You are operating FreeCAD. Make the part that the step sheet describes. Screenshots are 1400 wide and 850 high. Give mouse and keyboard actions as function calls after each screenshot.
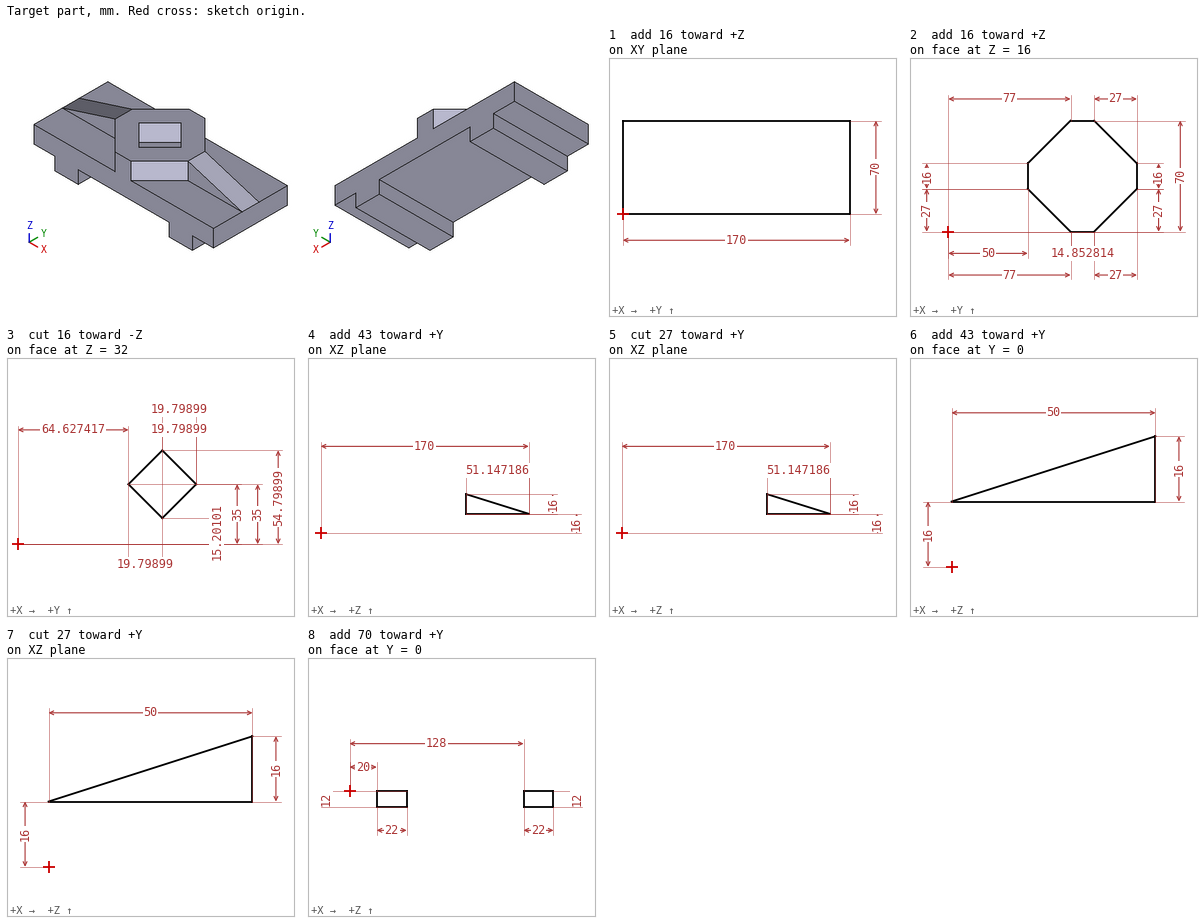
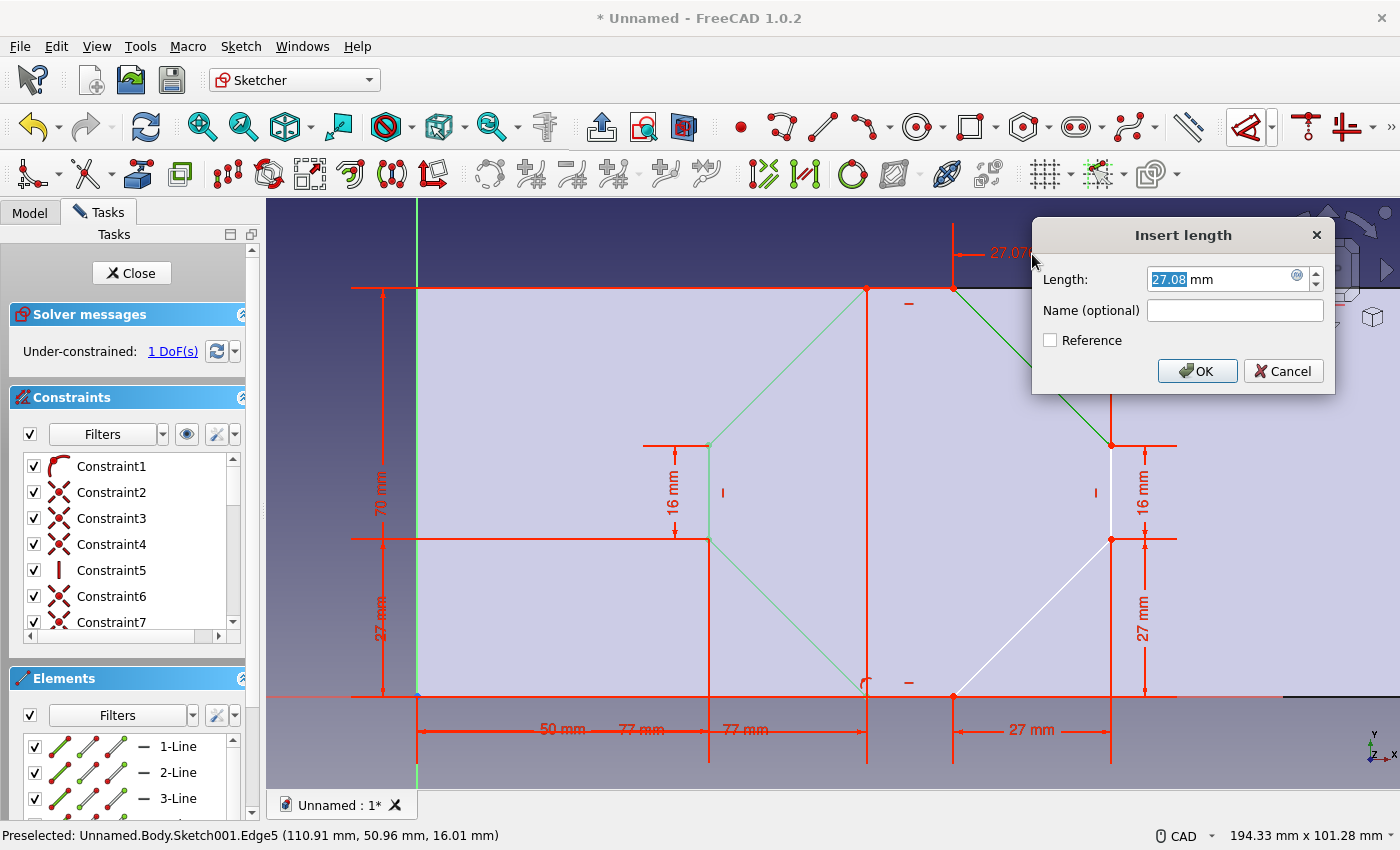
text(27)
key(Return)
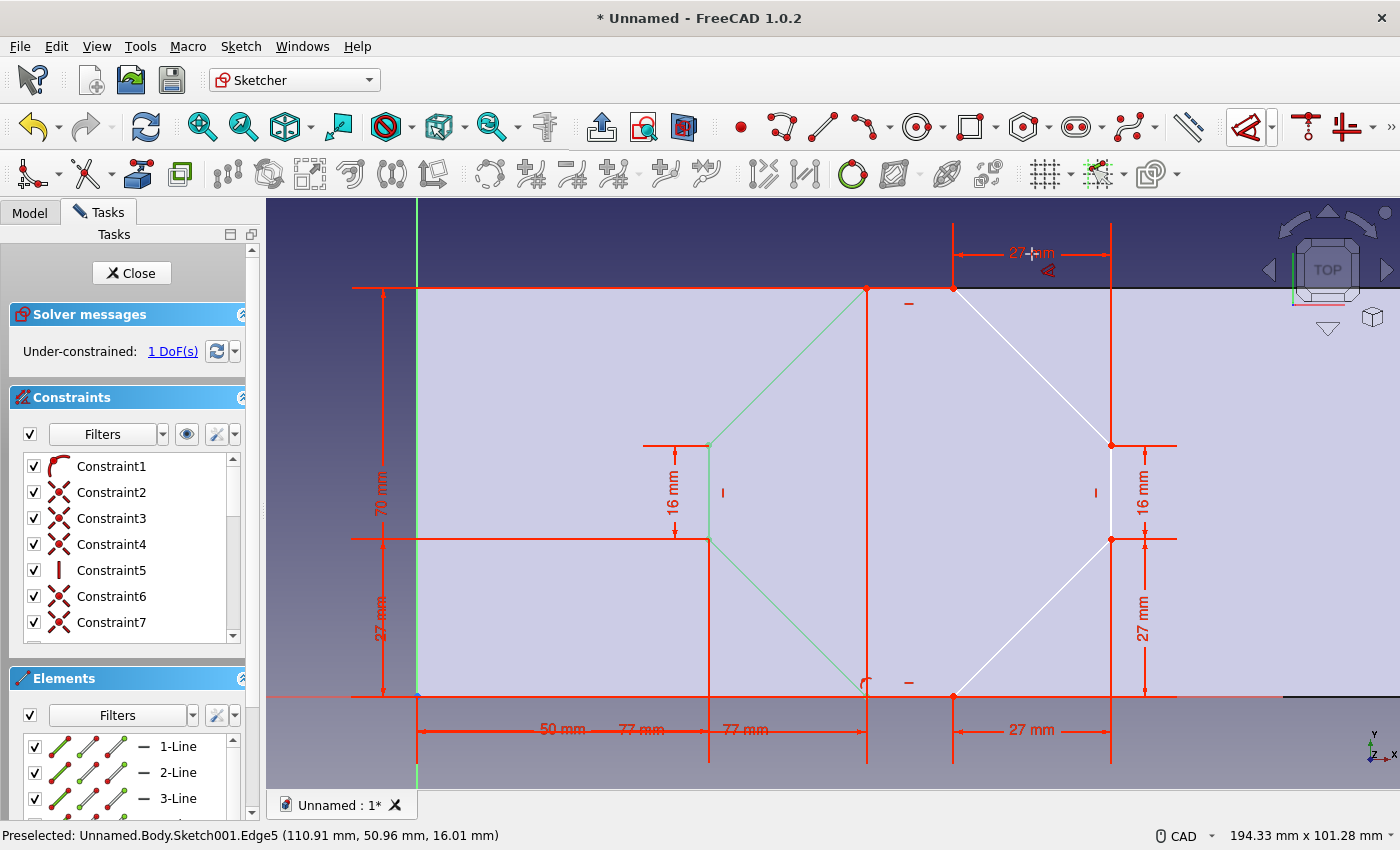
click(893, 697)
click(910, 731)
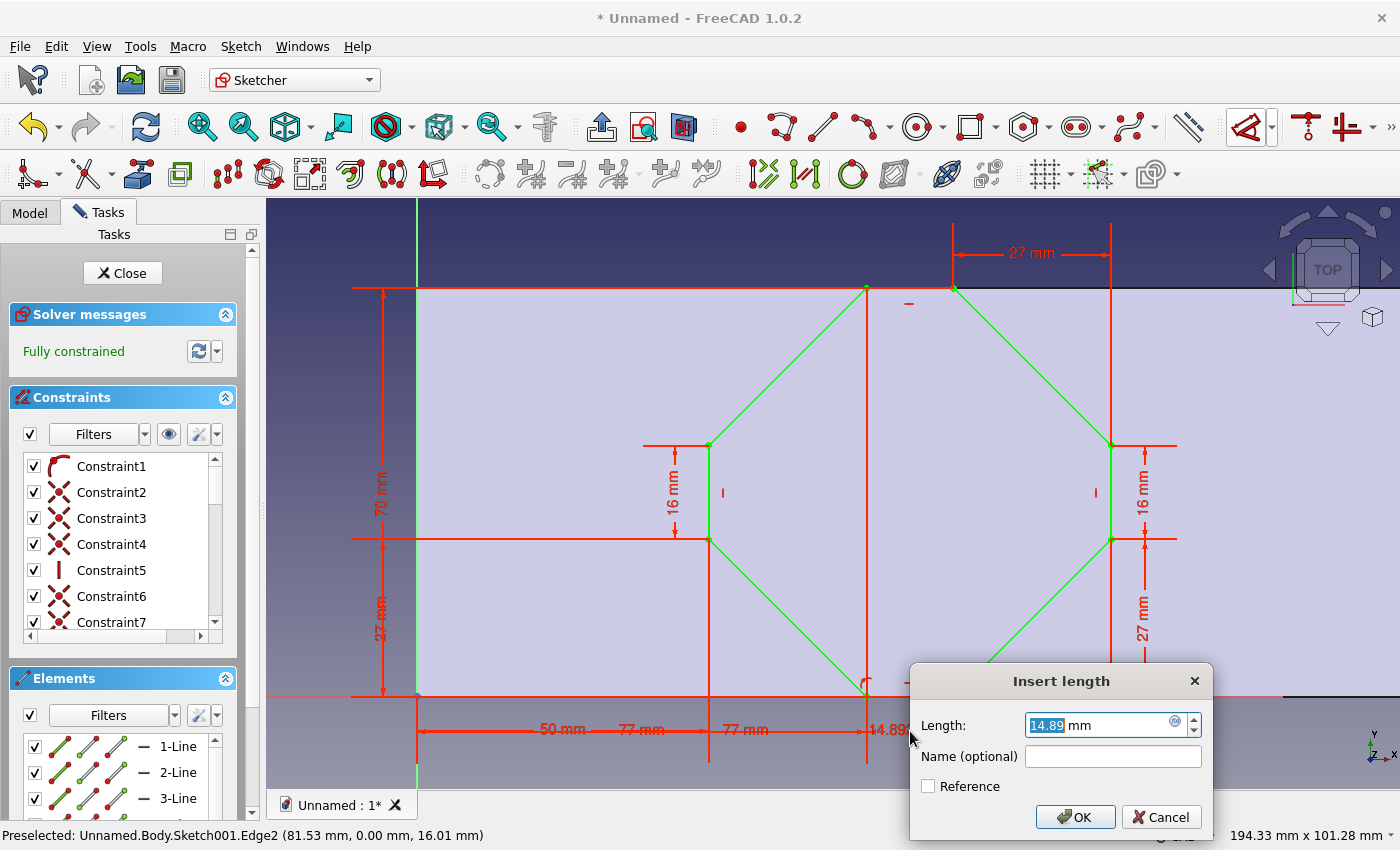
text(14.852814)
key(Return)
key(Escape)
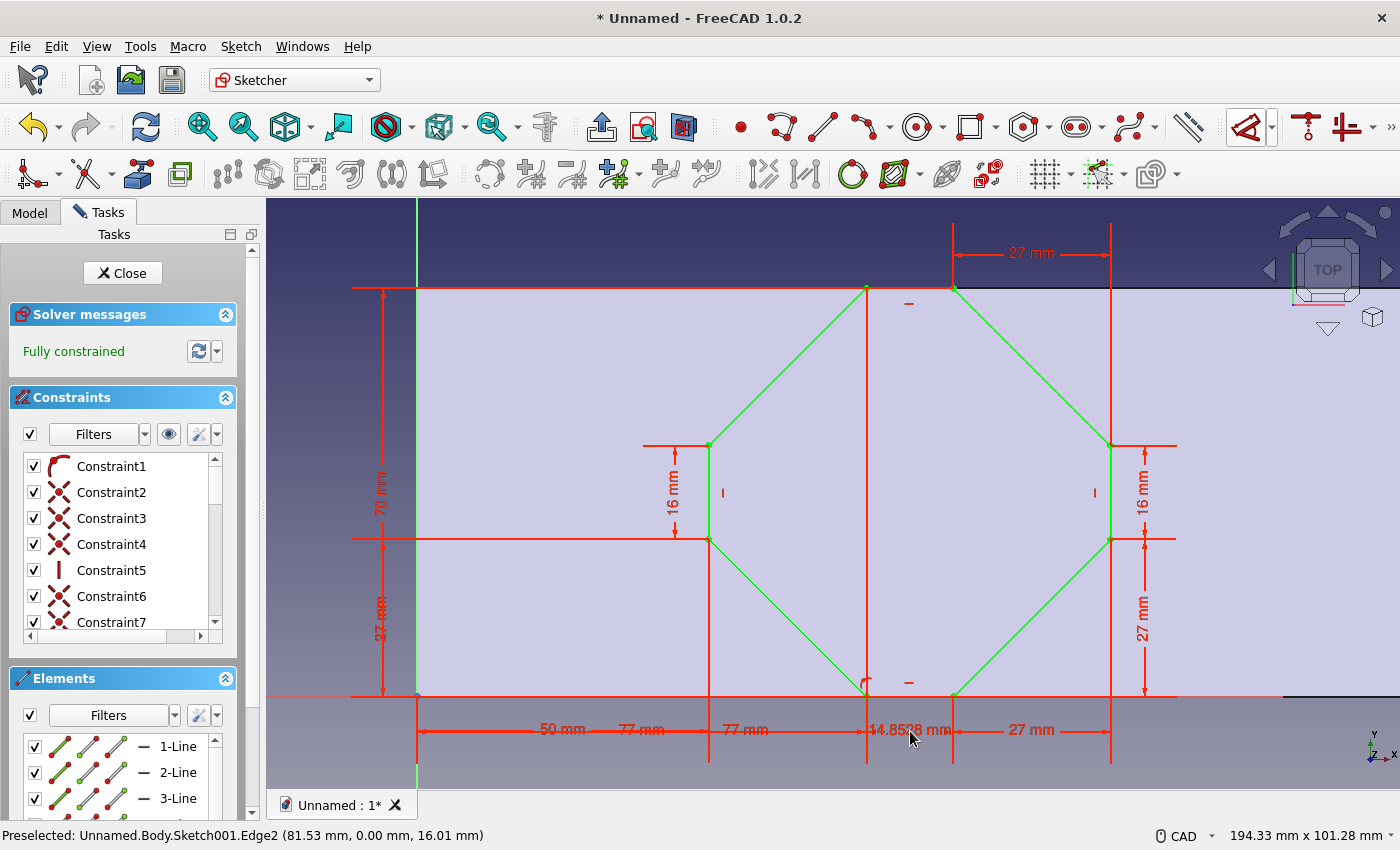
click(123, 273)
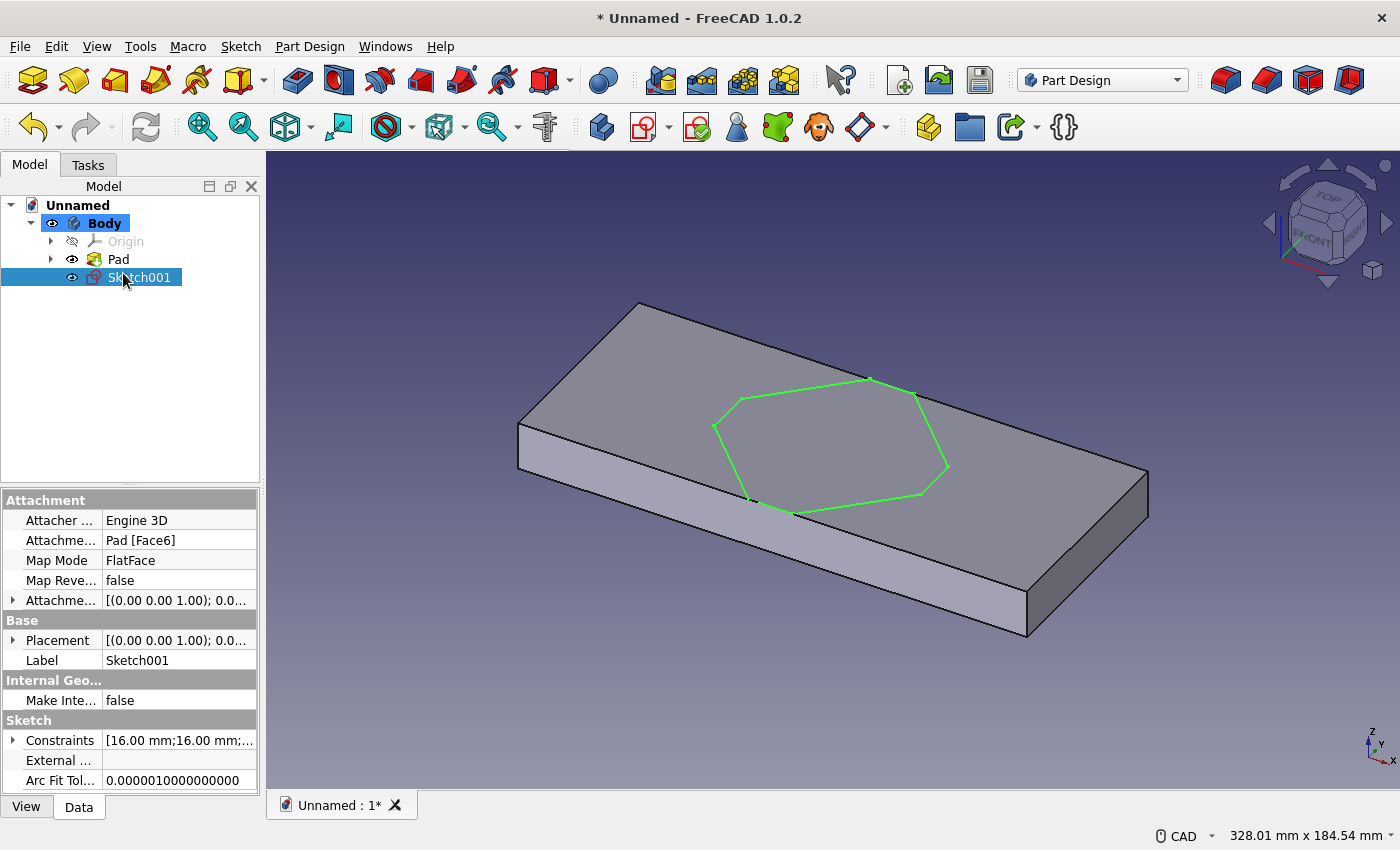
click(33, 80)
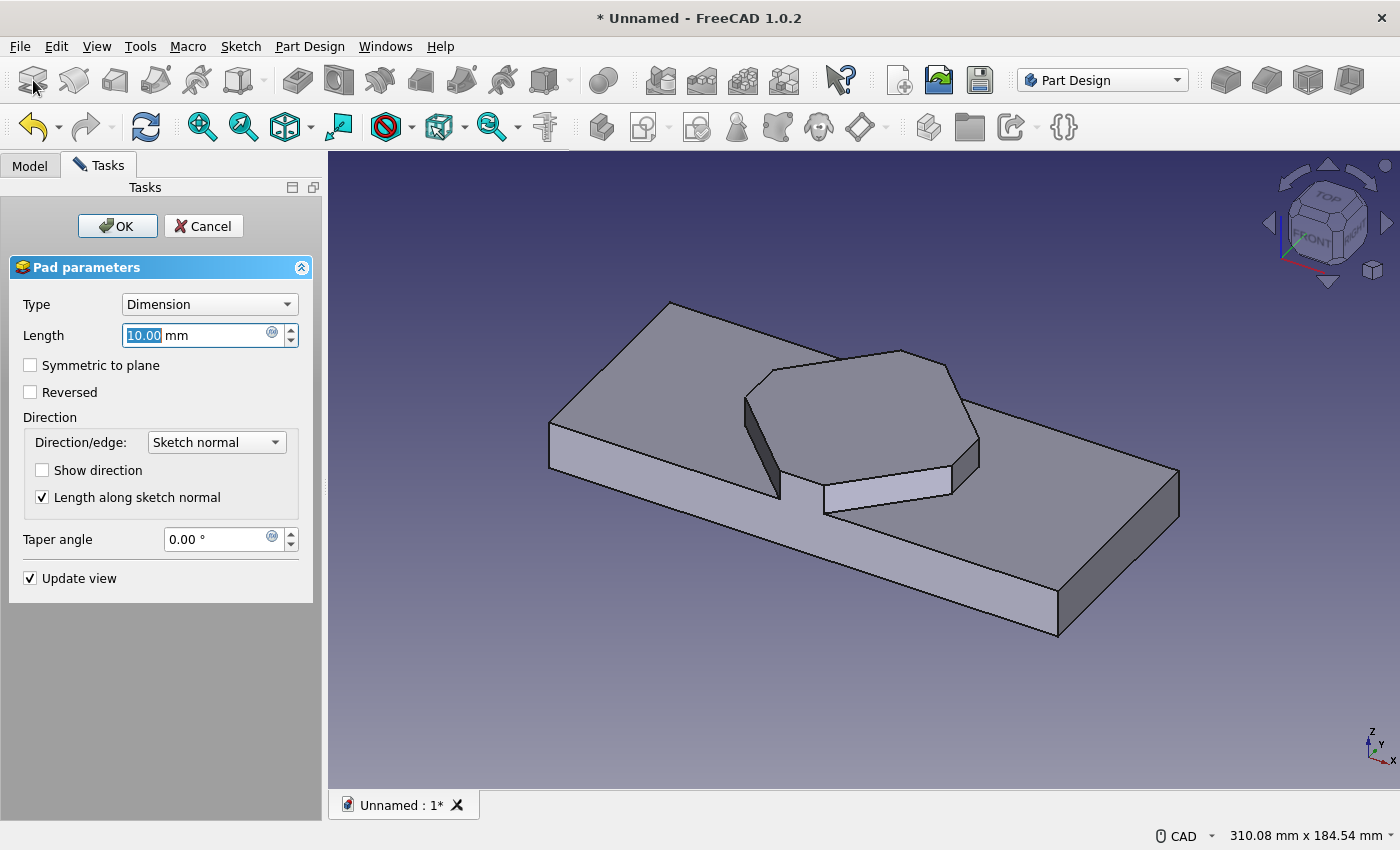
text(16)
key(Tab)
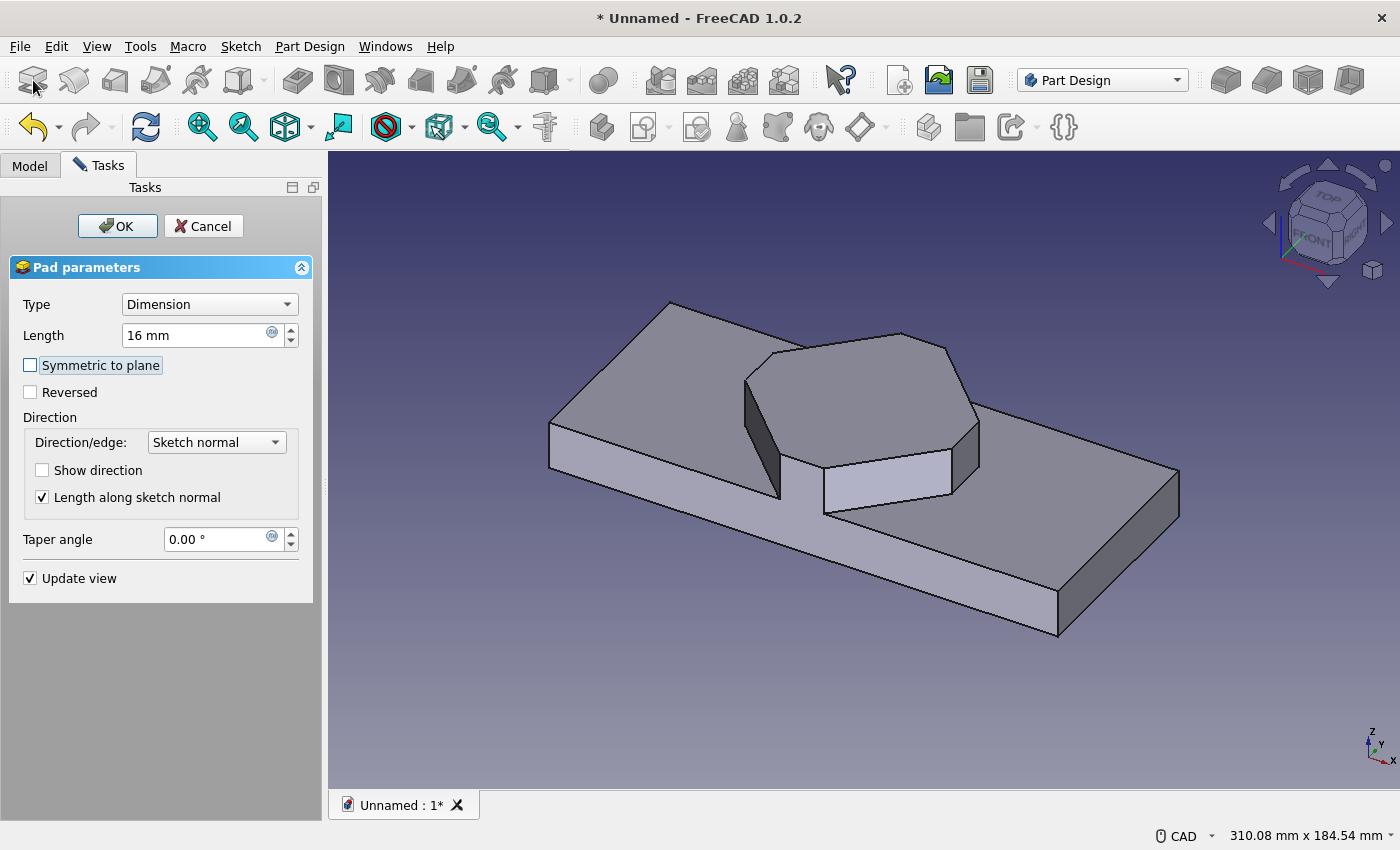
click(118, 226)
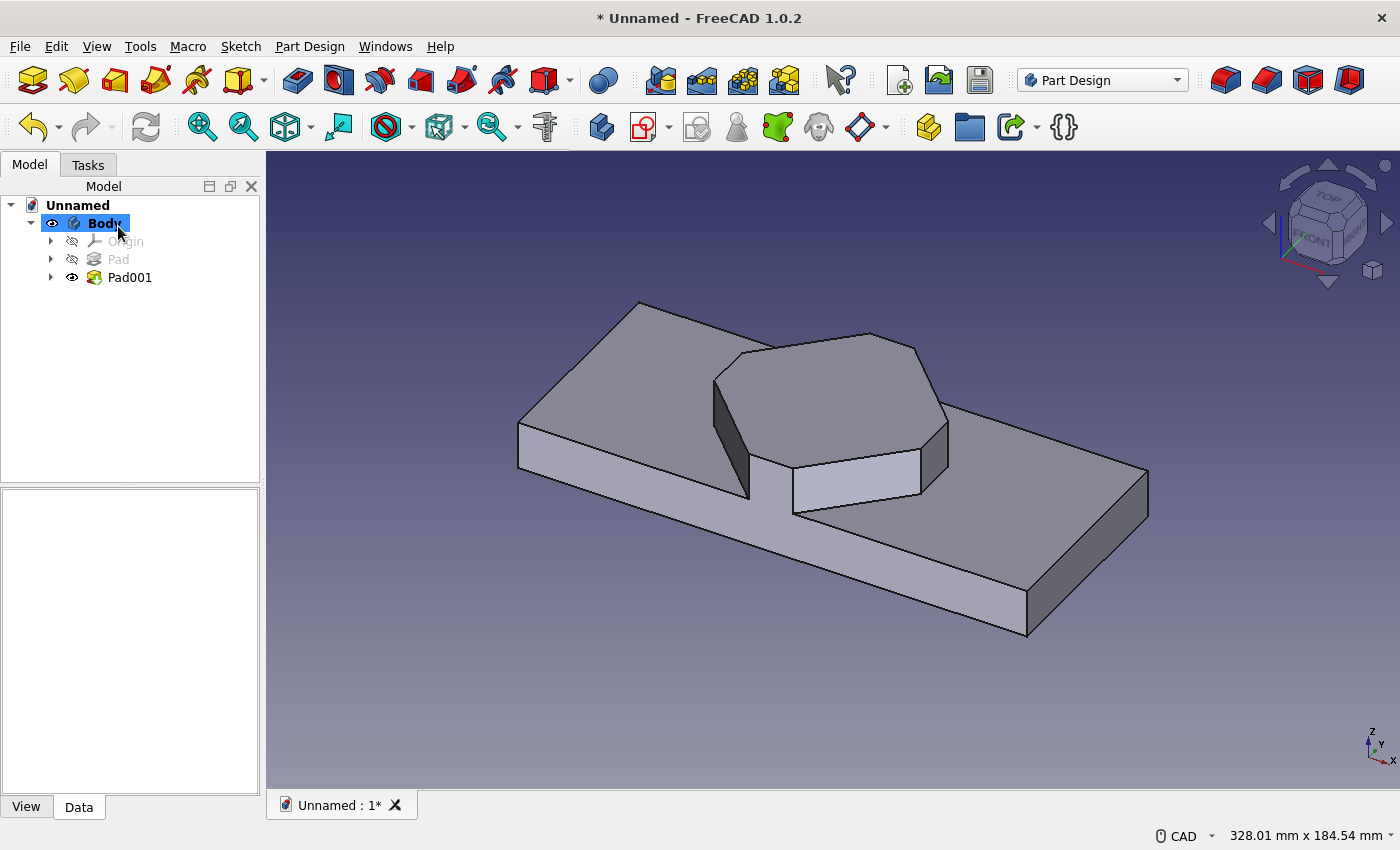
click(831, 400)